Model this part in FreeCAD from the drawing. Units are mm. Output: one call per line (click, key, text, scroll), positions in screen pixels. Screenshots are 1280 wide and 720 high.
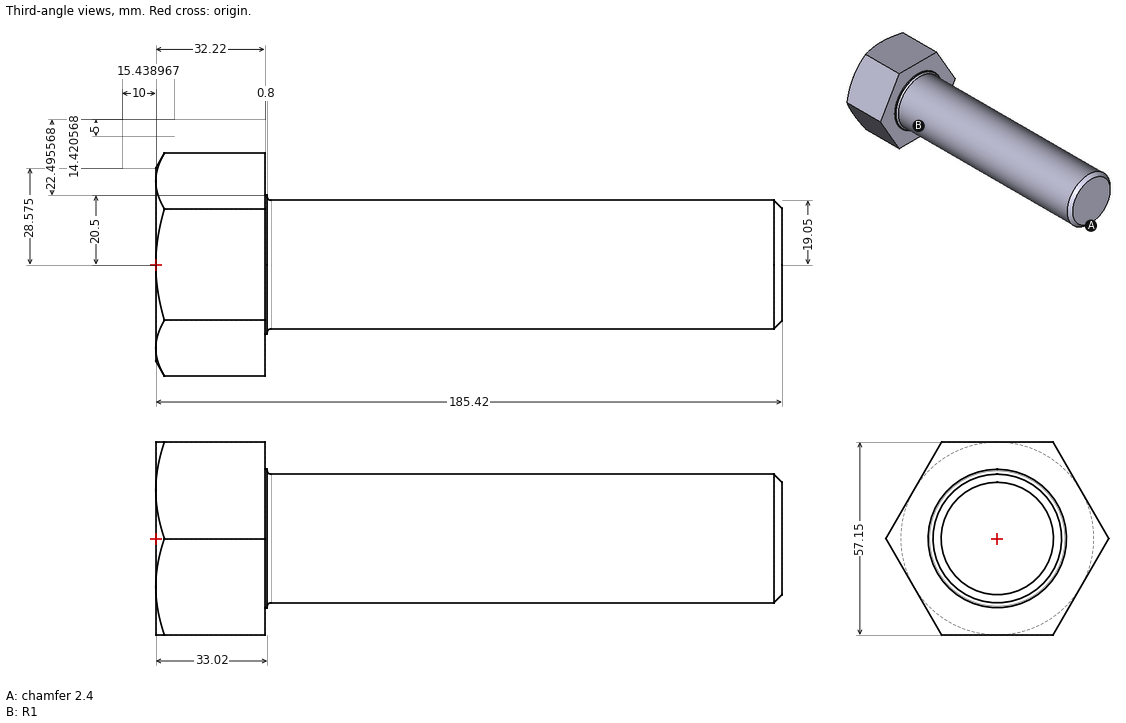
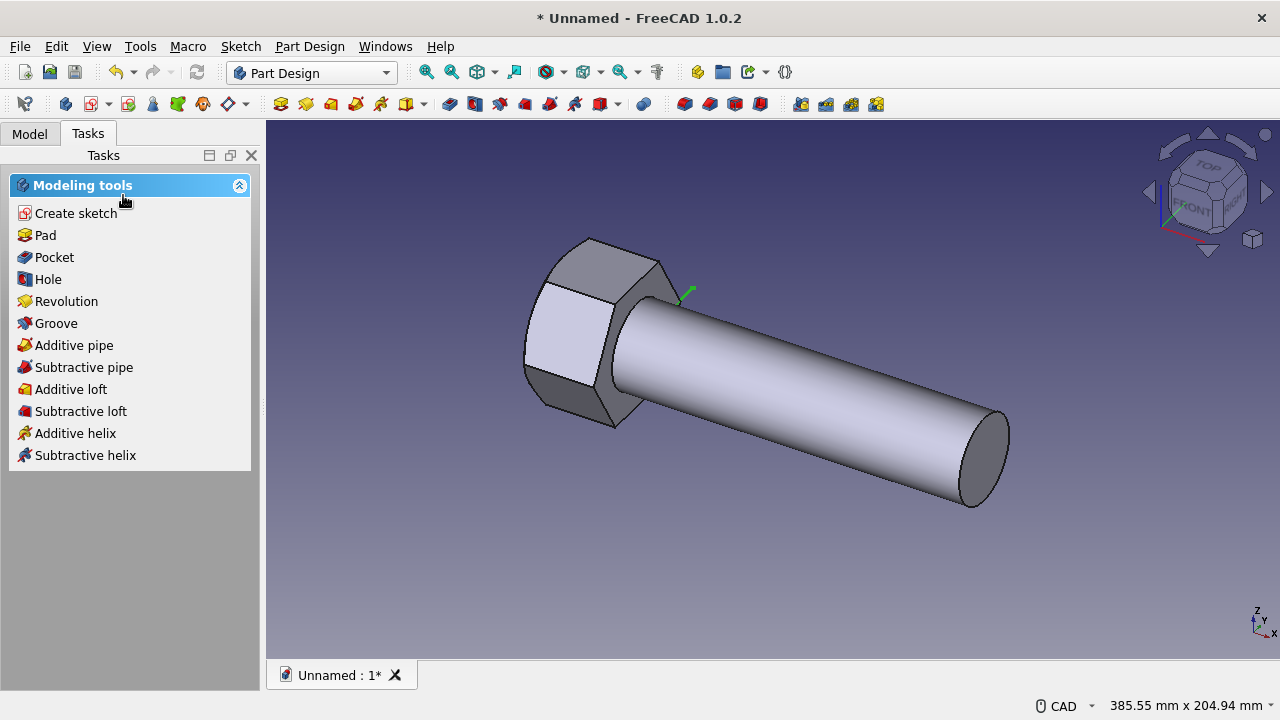
click(500, 104)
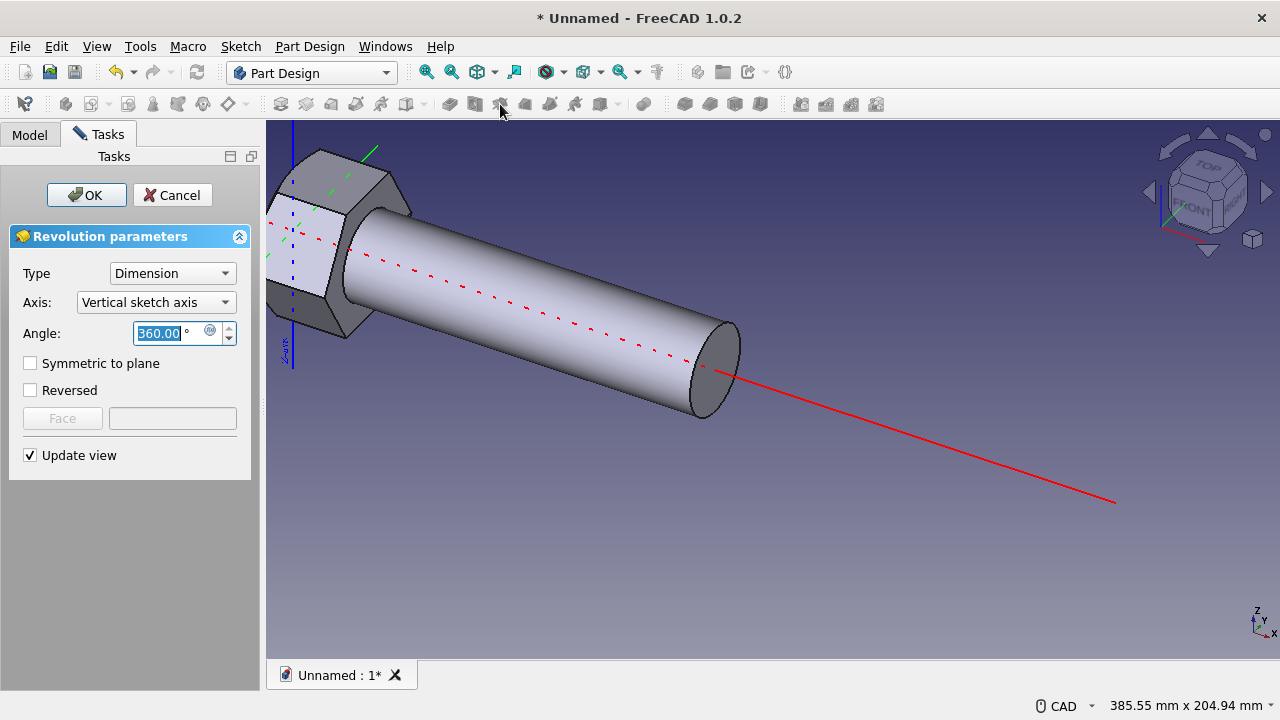
click(157, 302)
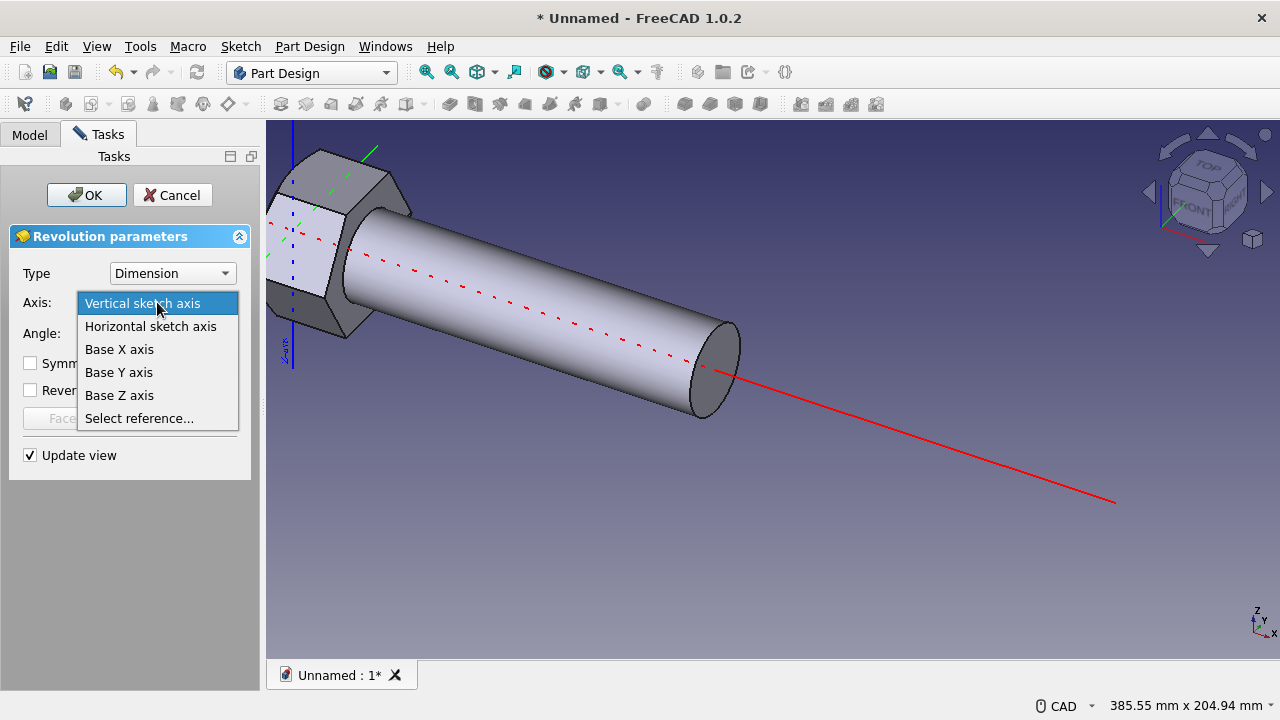
click(156, 326)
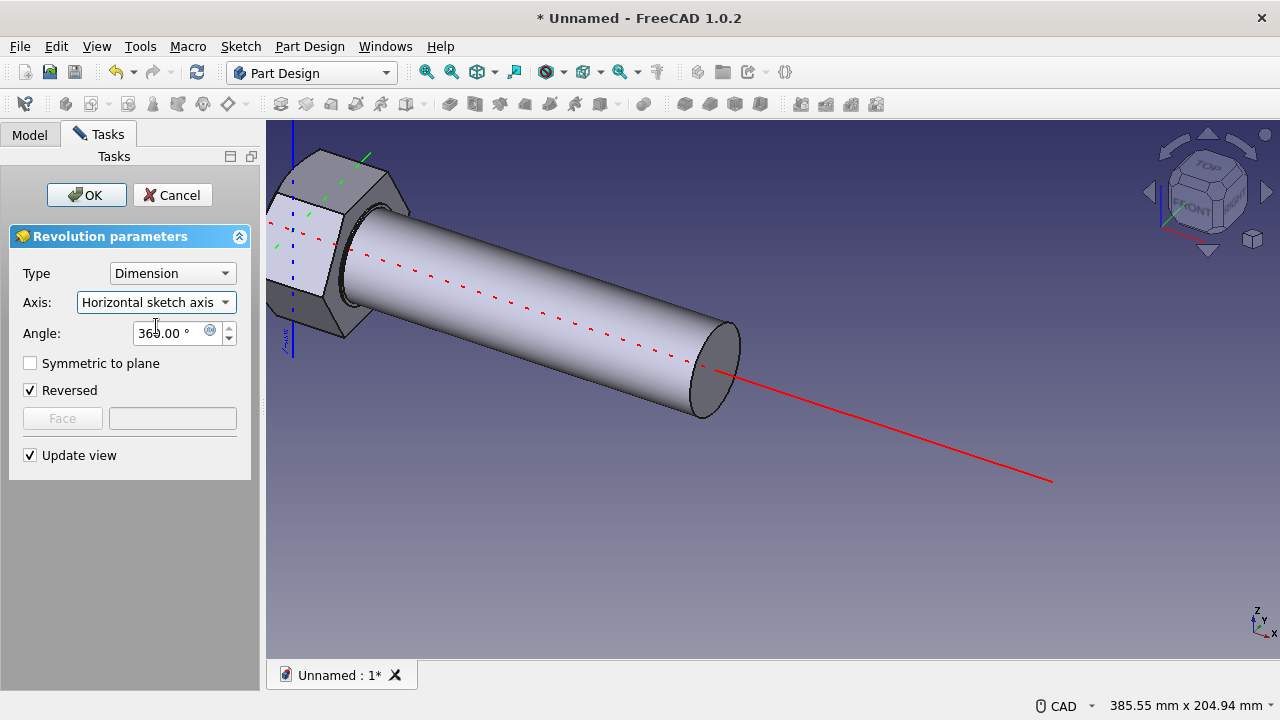
click(87, 195)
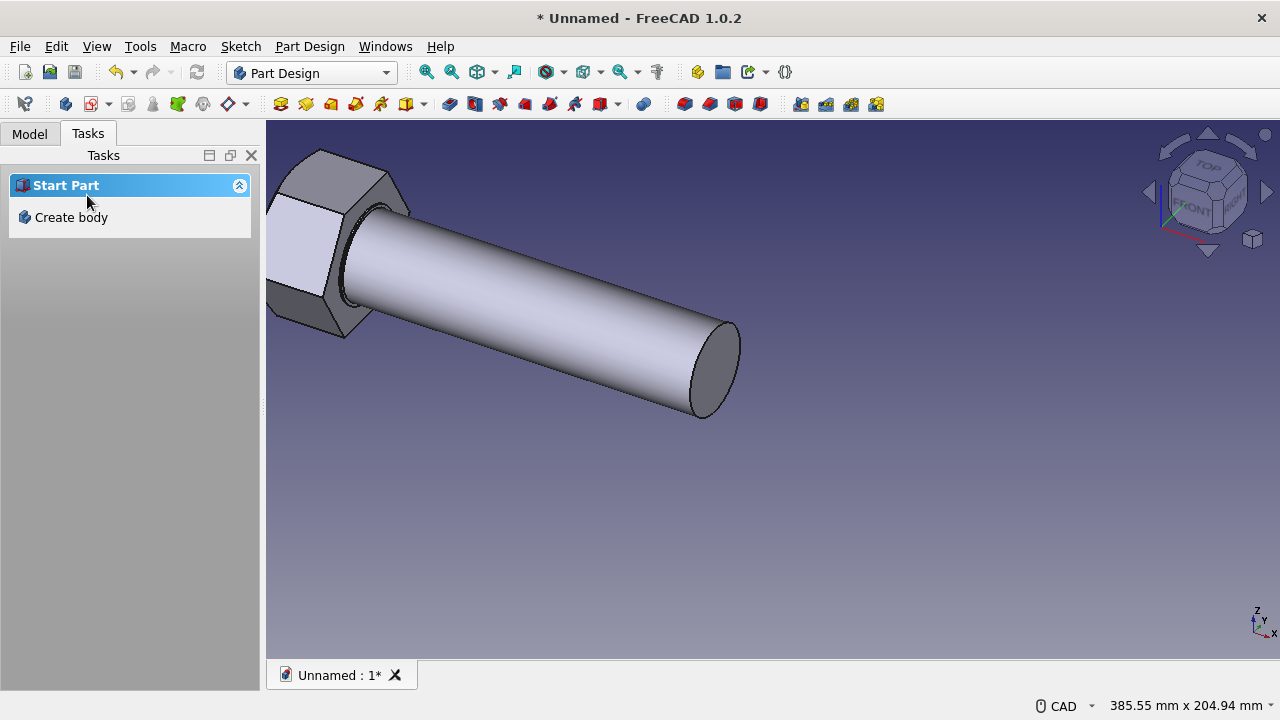
click(427, 72)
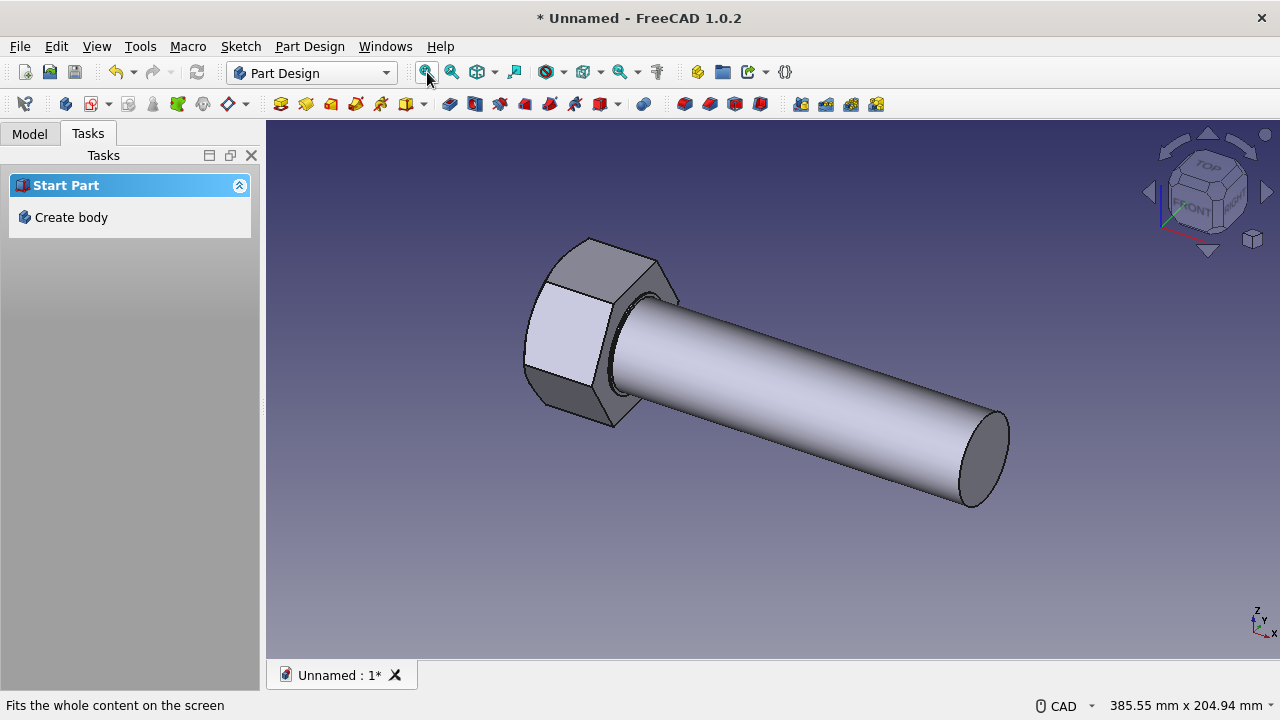
click(959, 483)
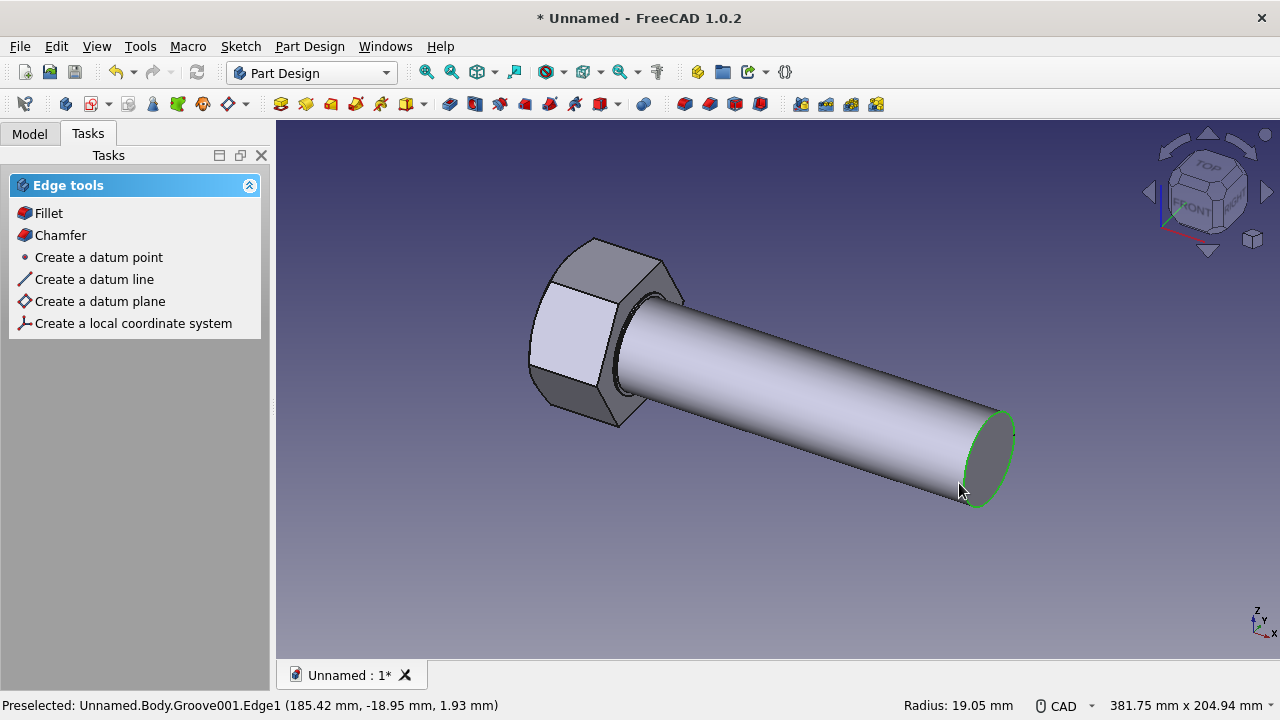
click(710, 104)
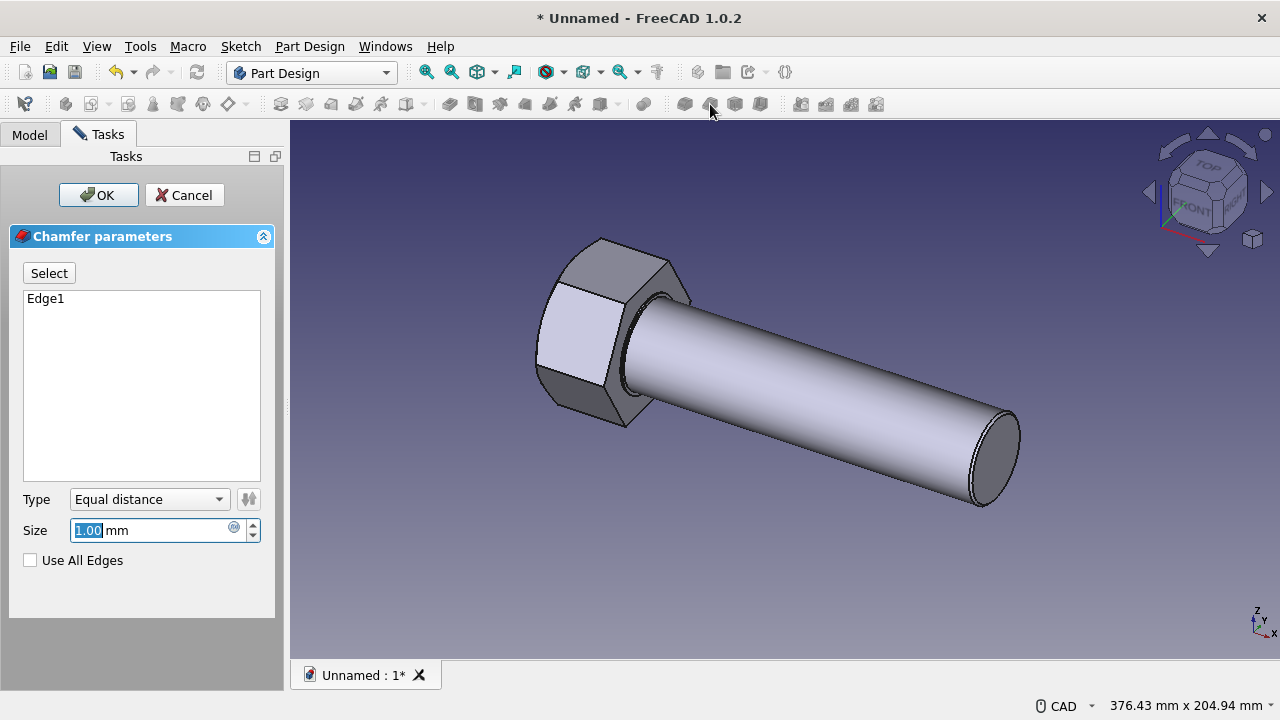
text(2.4)
key(Tab)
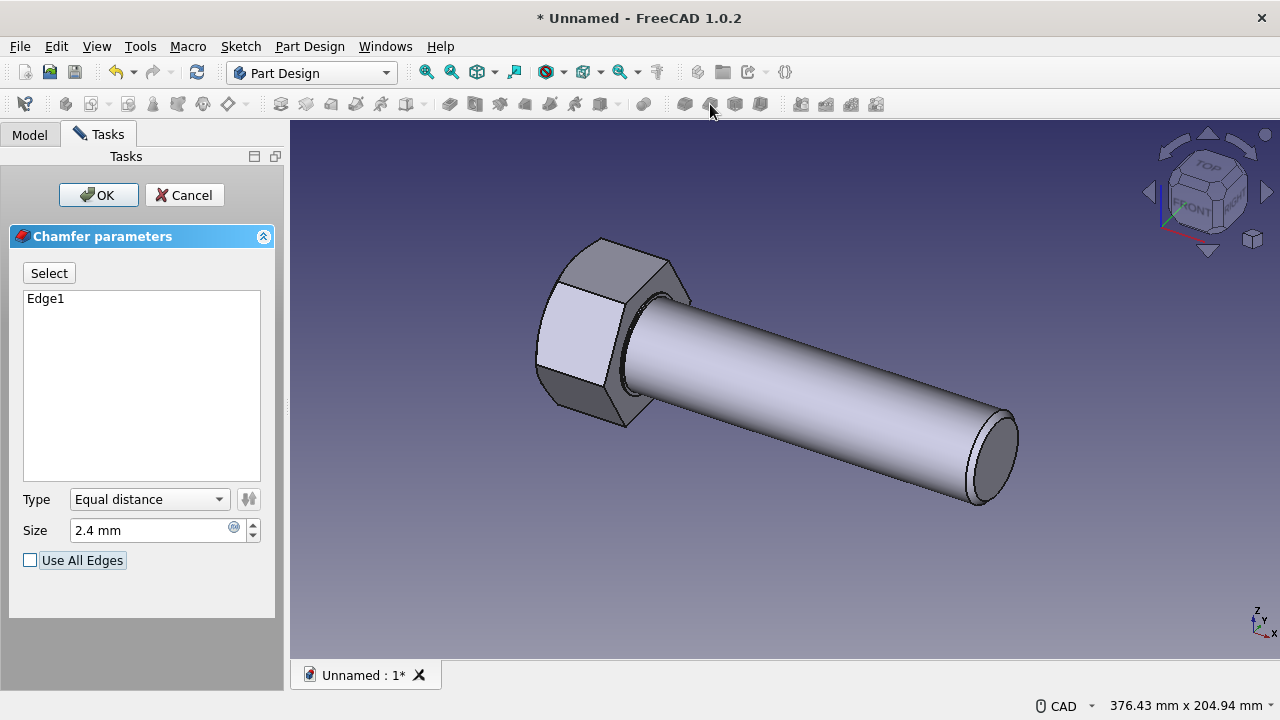
click(99, 195)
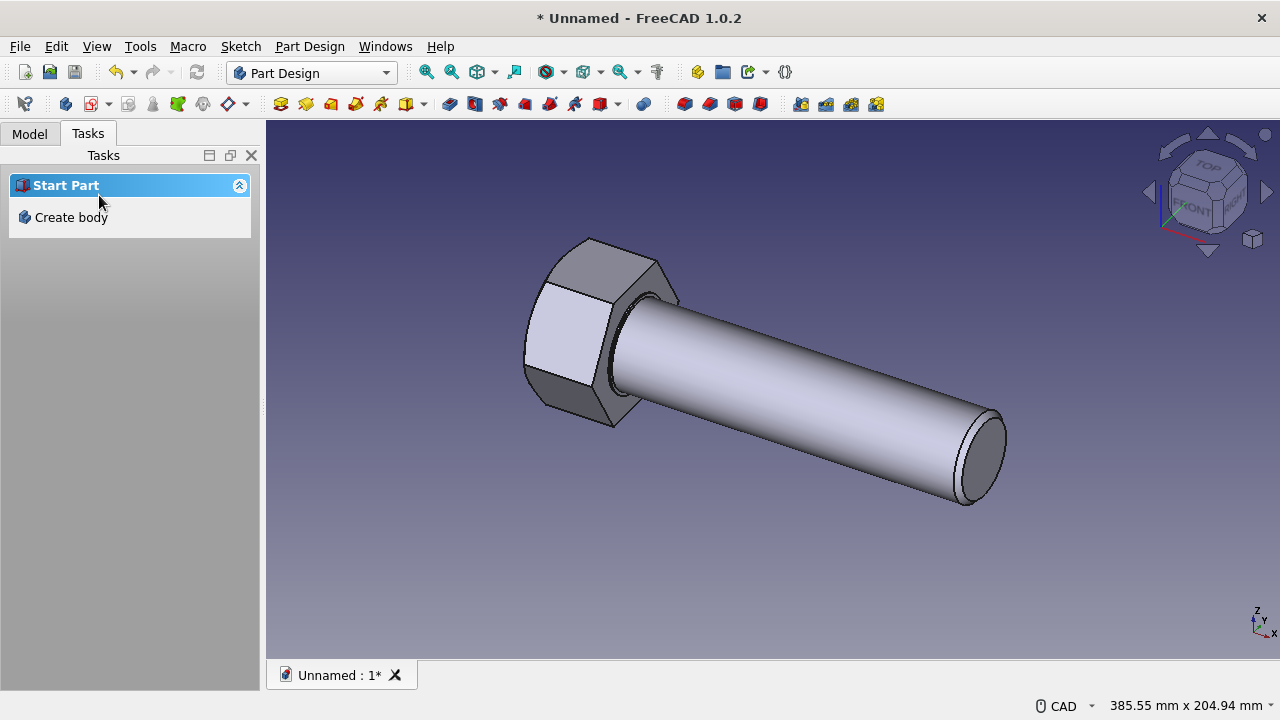
key(0)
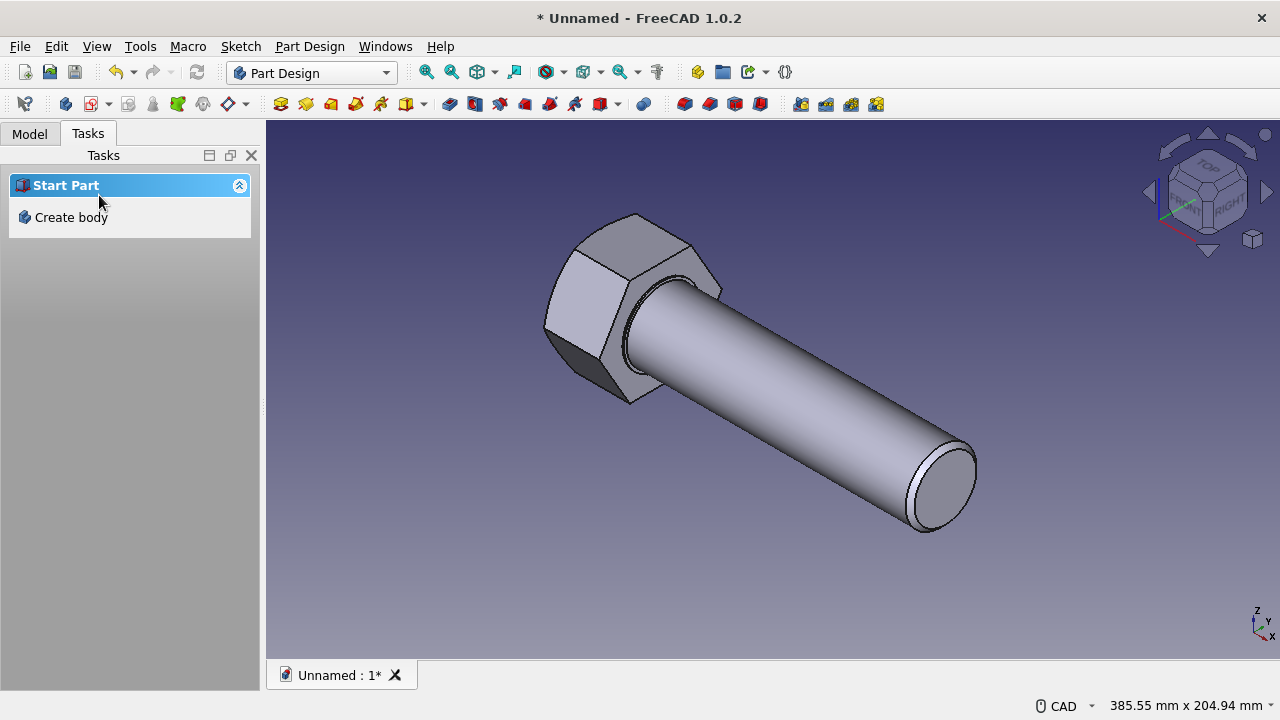
key(2)